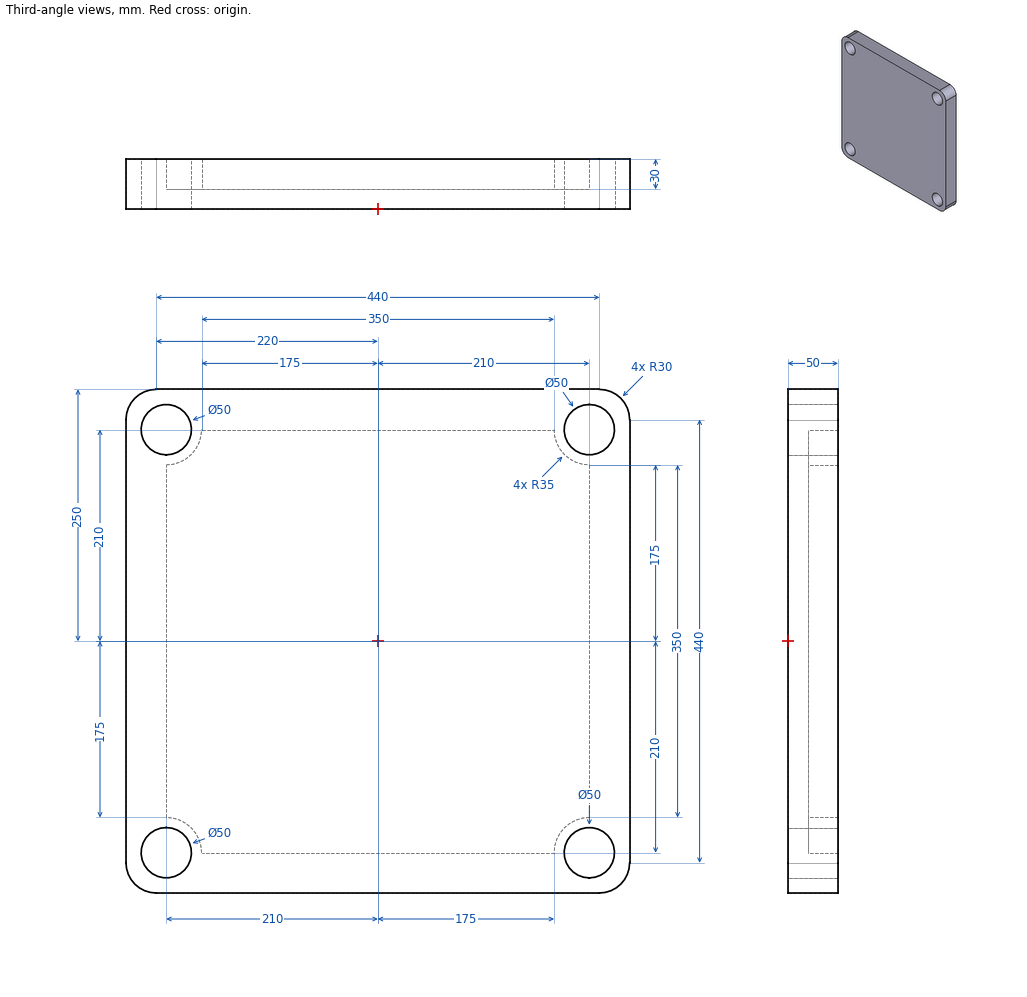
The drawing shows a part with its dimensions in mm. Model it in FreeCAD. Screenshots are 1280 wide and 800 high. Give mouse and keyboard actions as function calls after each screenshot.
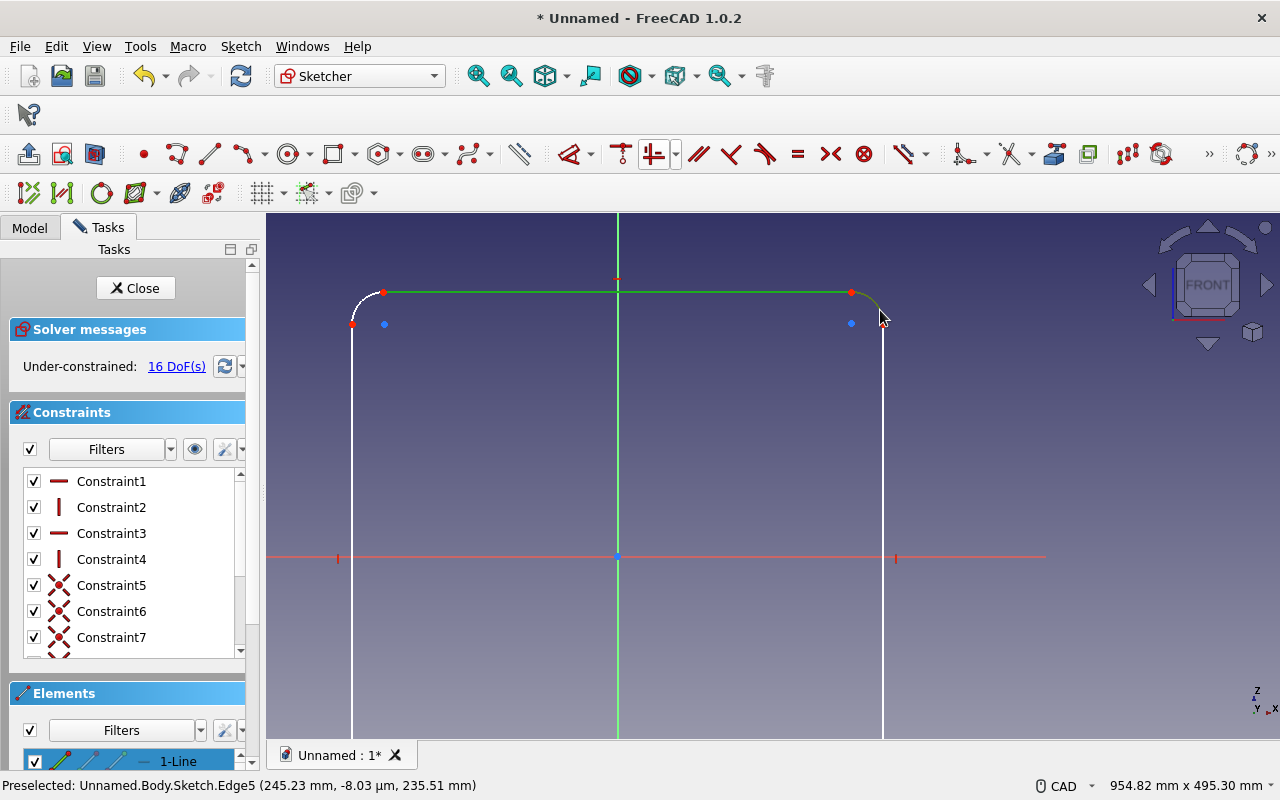
click(765, 154)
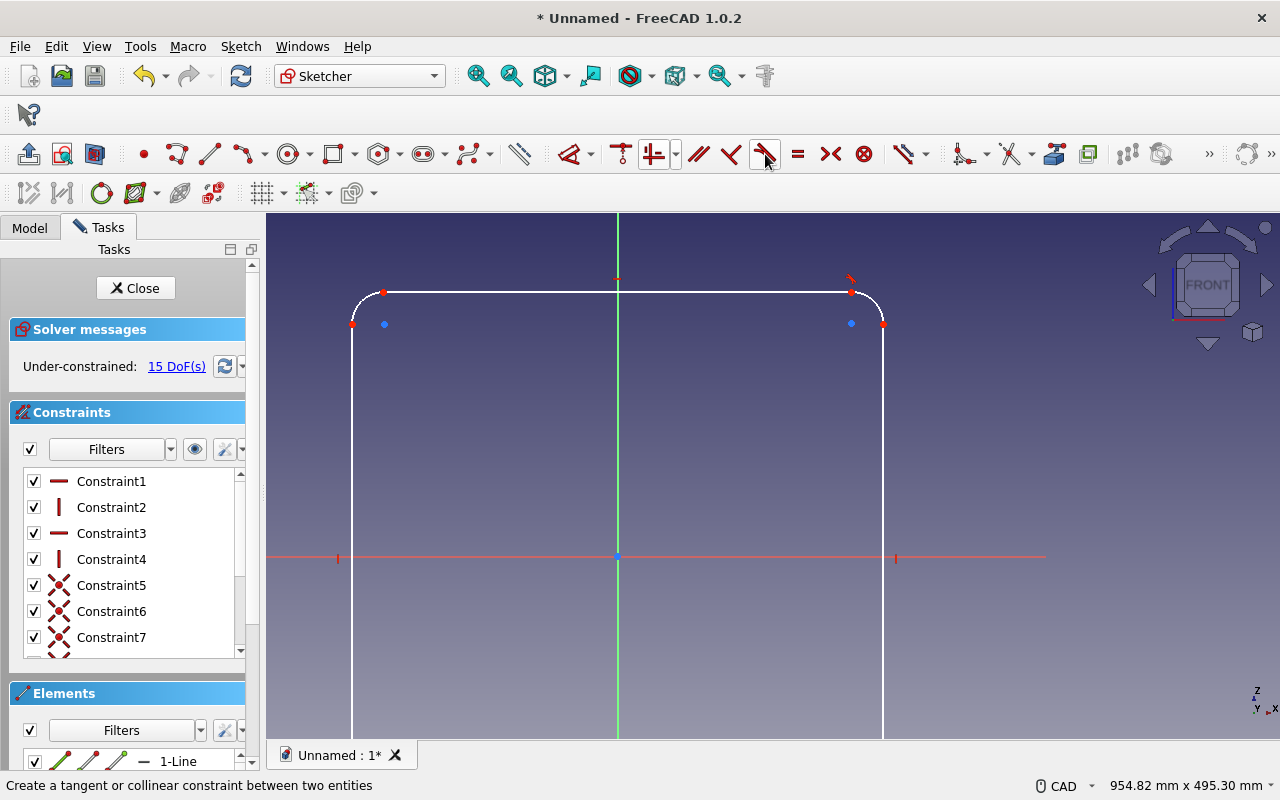
click(524, 292)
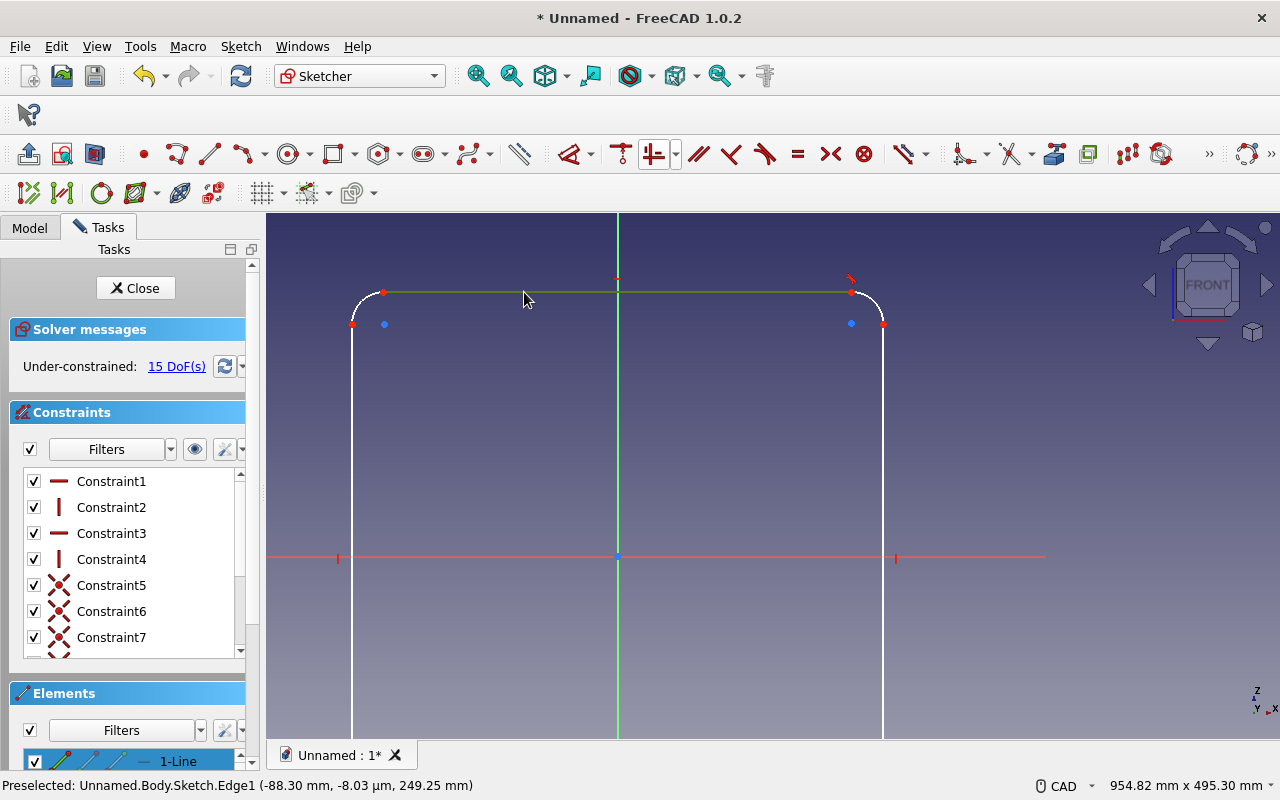
click(369, 296)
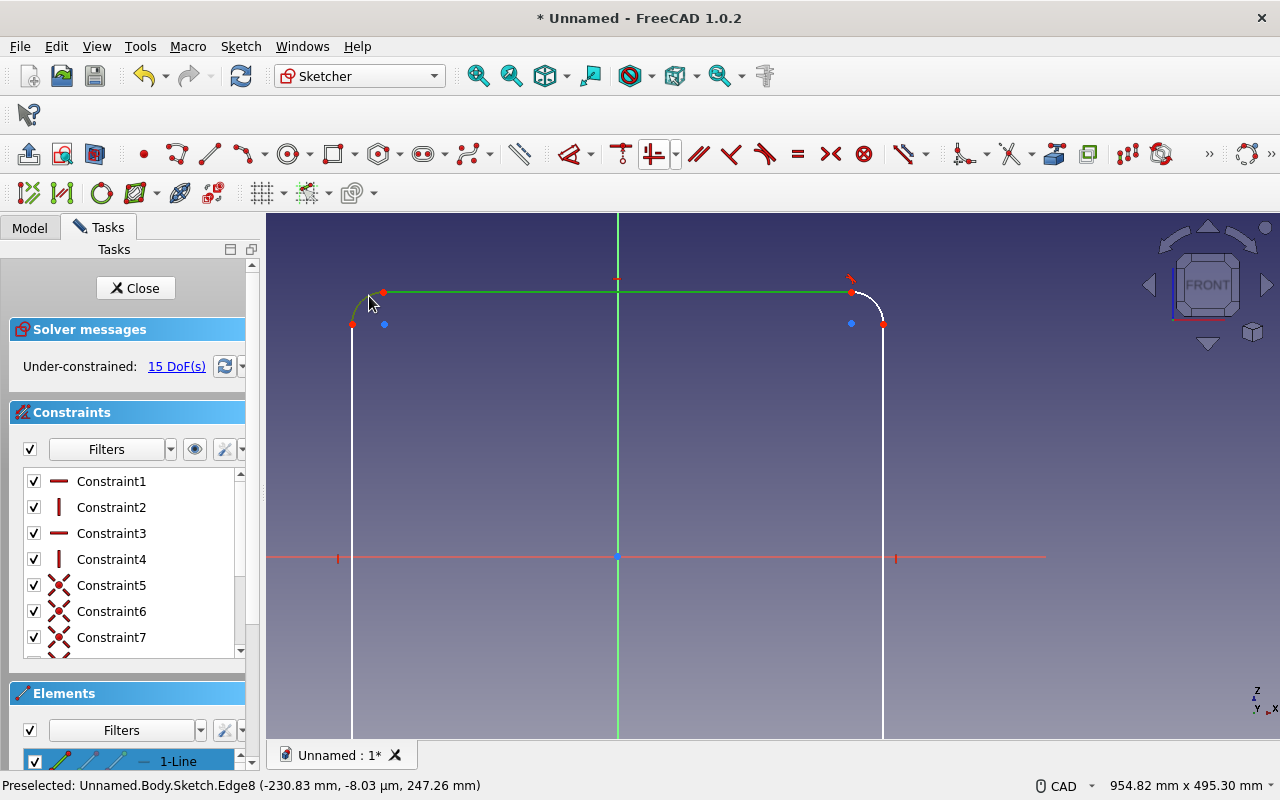
click(765, 154)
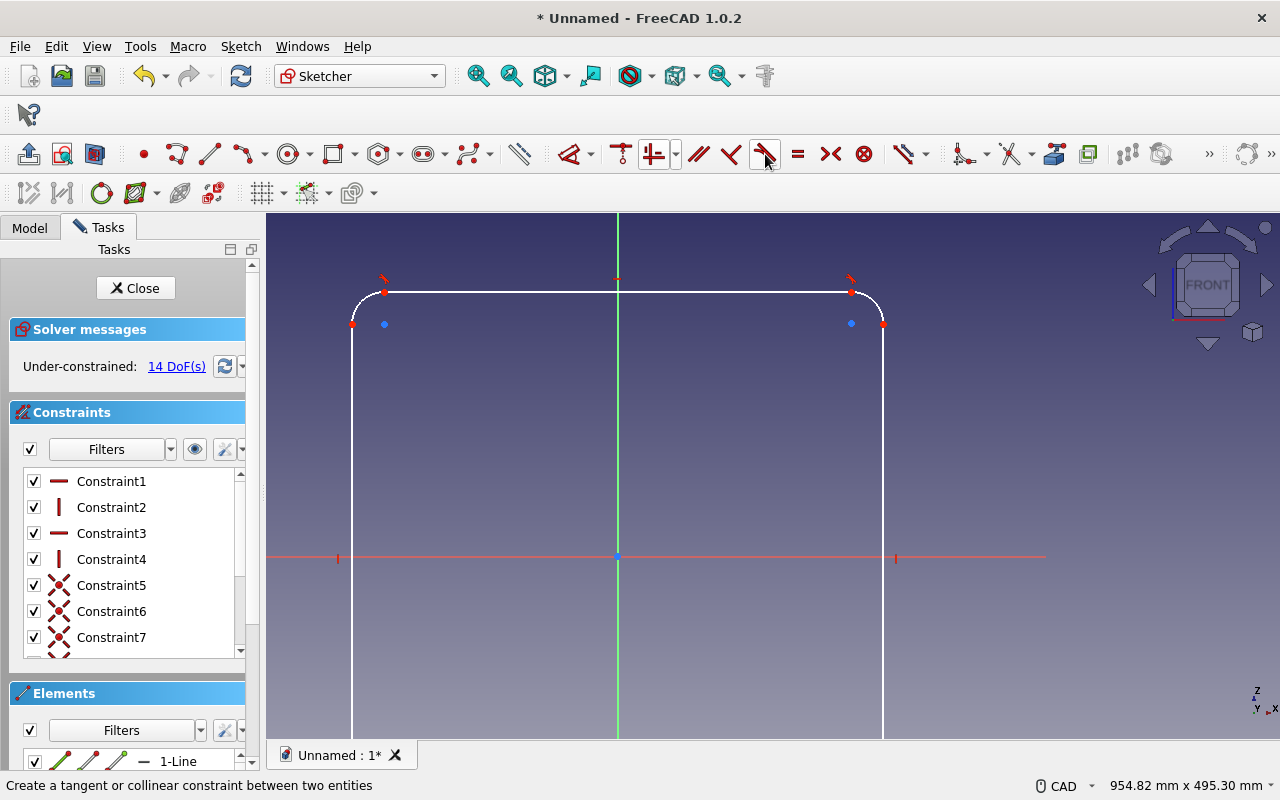
click(883, 465)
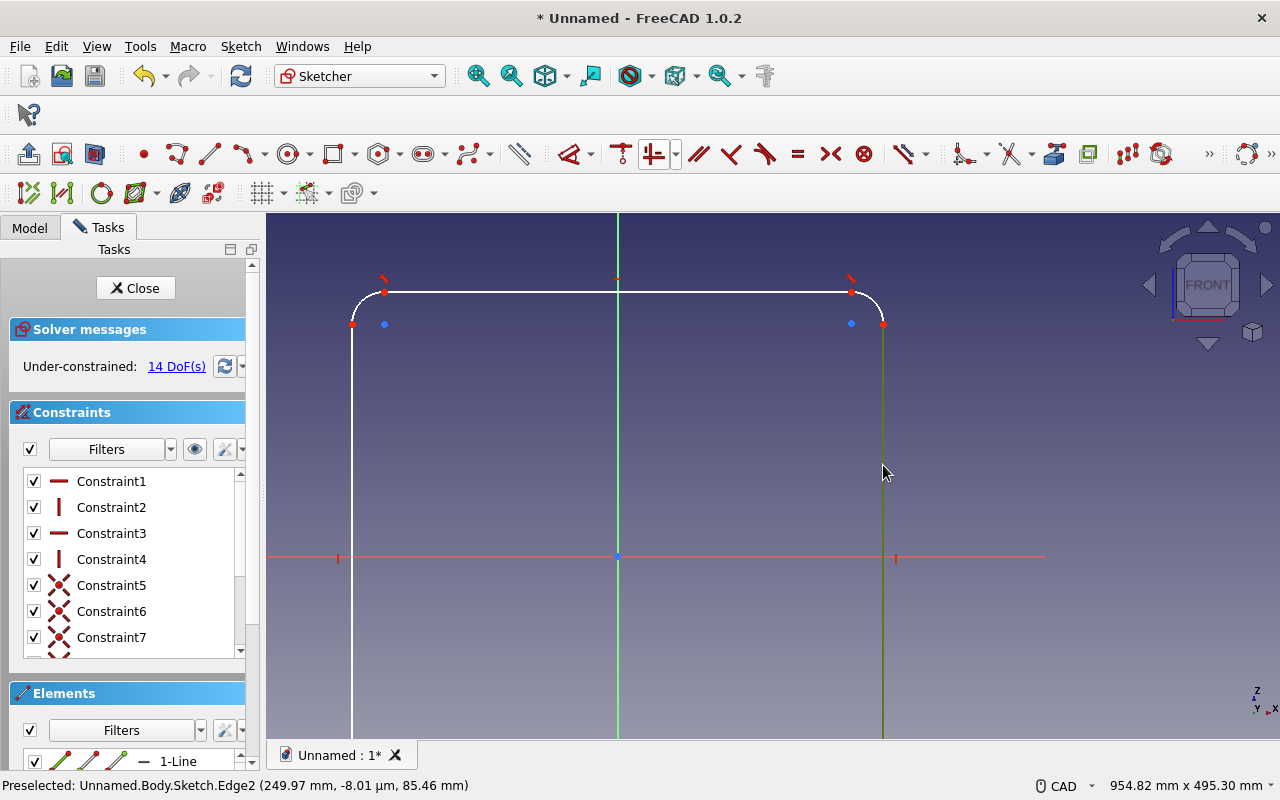
click(880, 310)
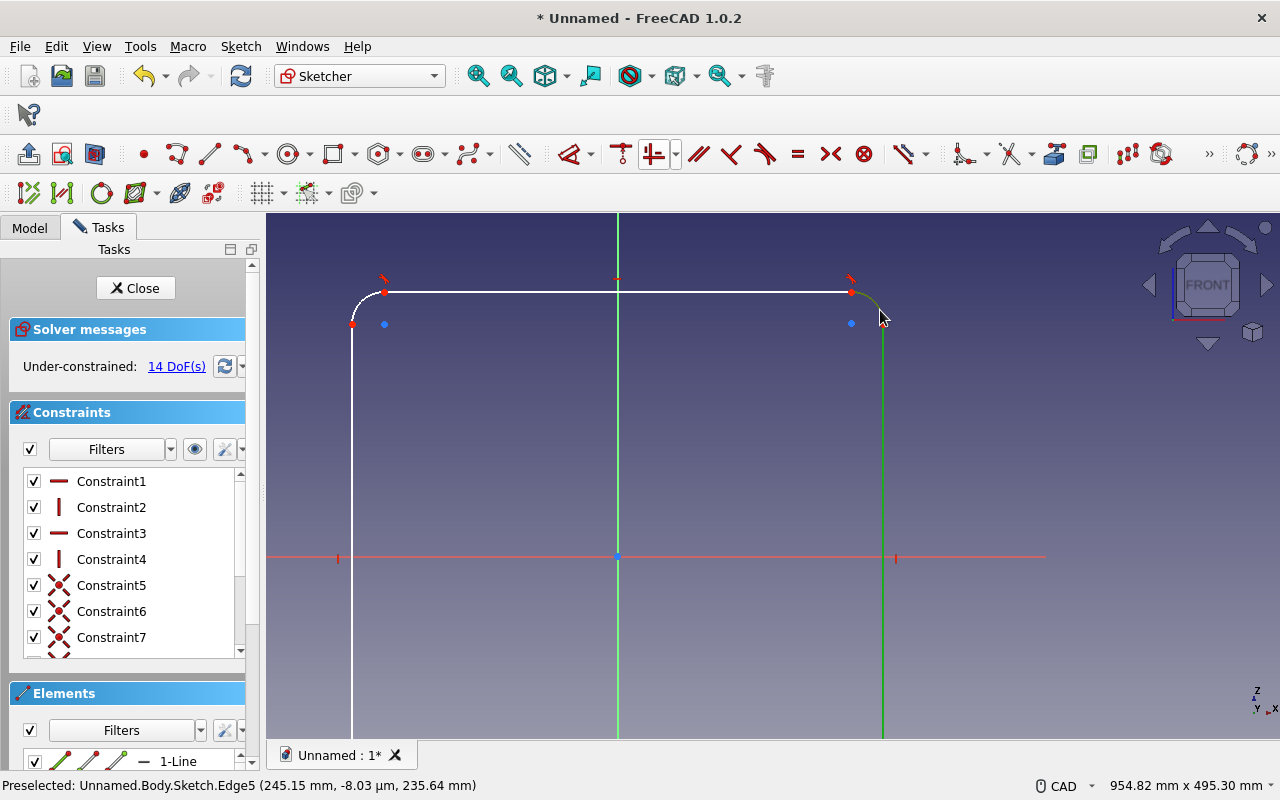
click(765, 154)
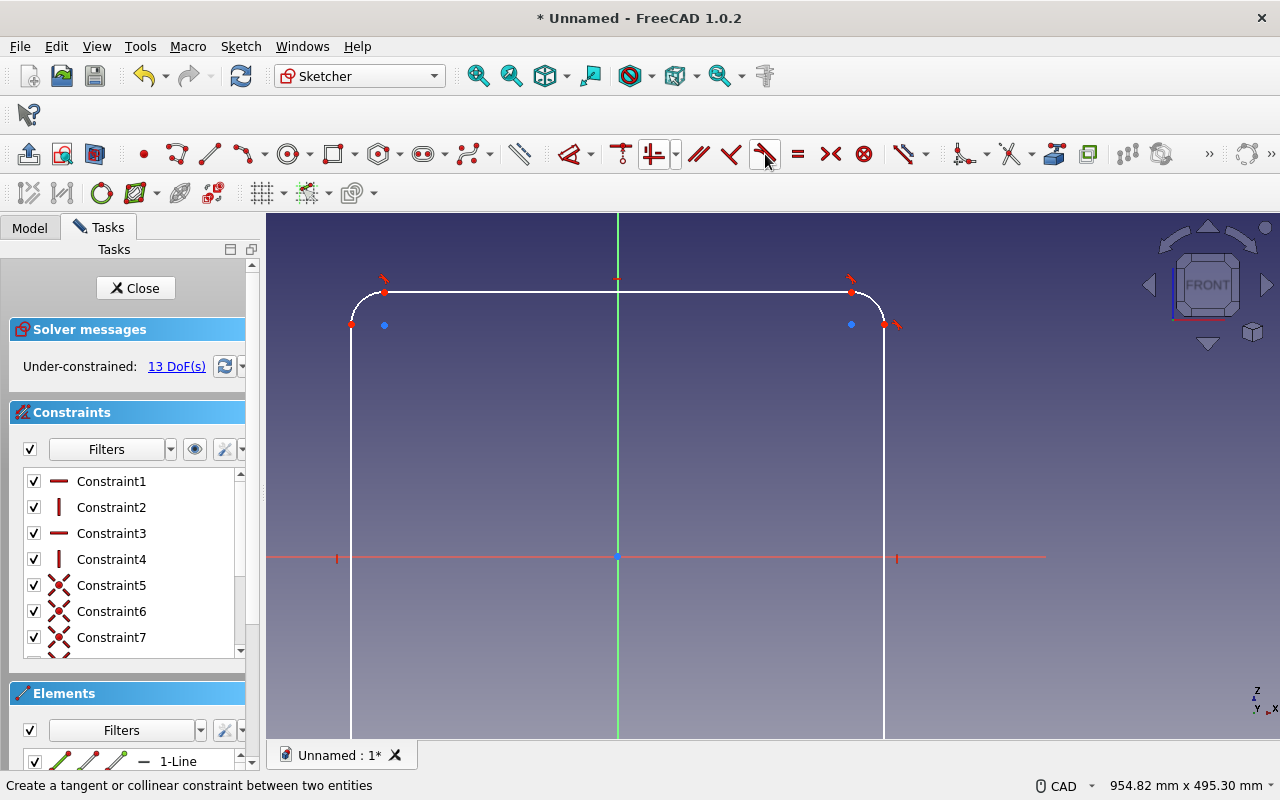
click(884, 465)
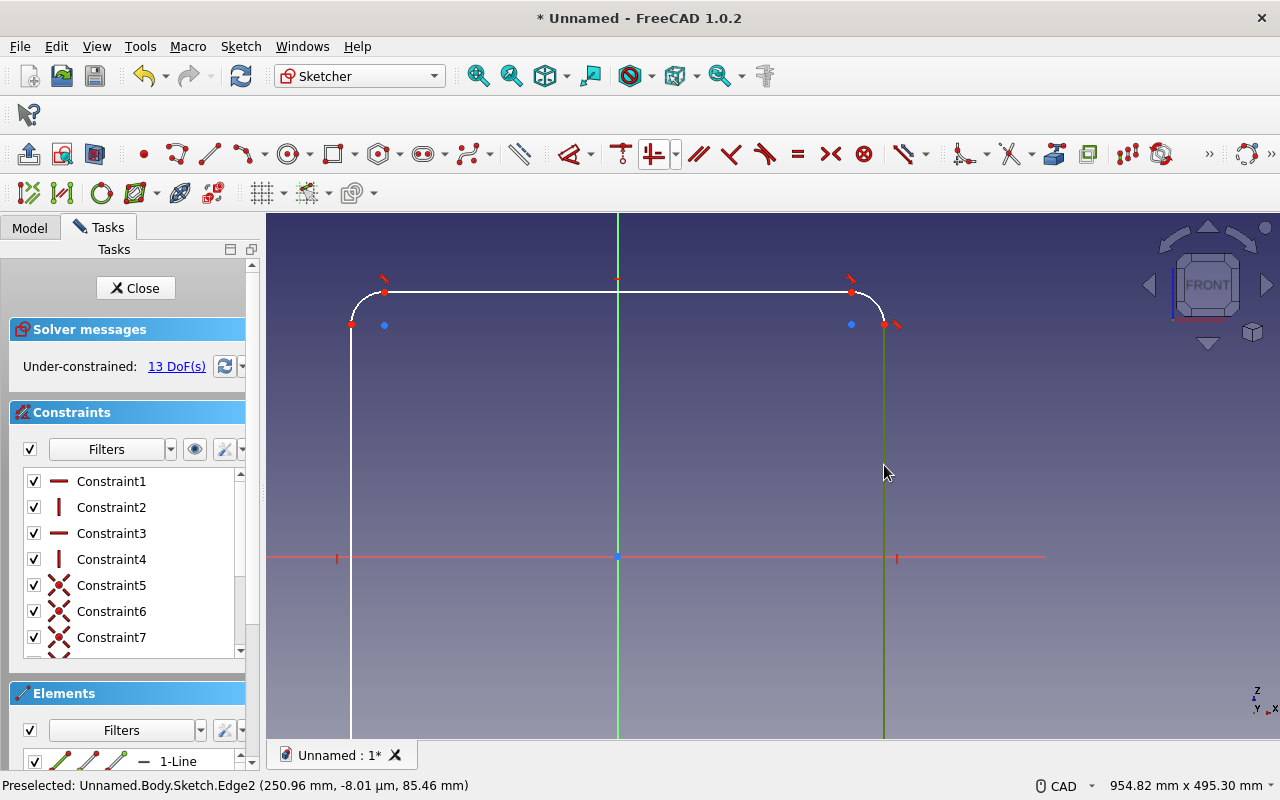
scroll(881, 312, down, 2)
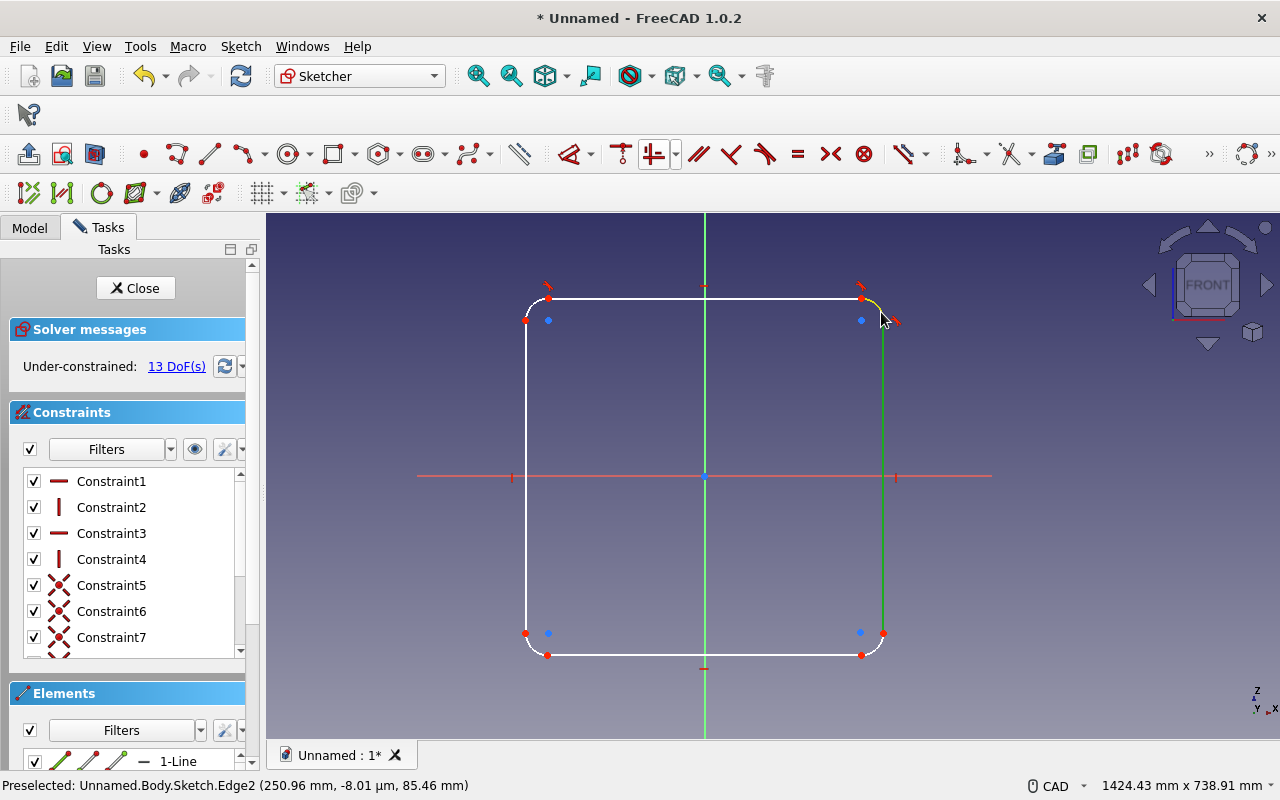
scroll(871, 653, up, 2)